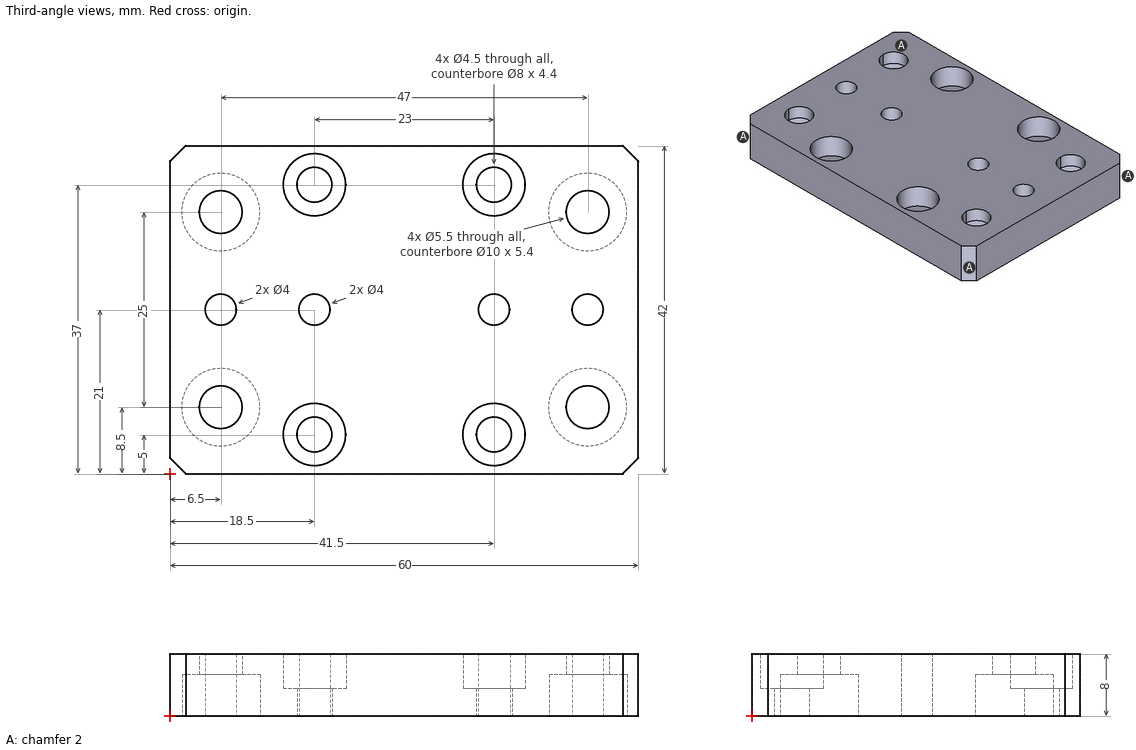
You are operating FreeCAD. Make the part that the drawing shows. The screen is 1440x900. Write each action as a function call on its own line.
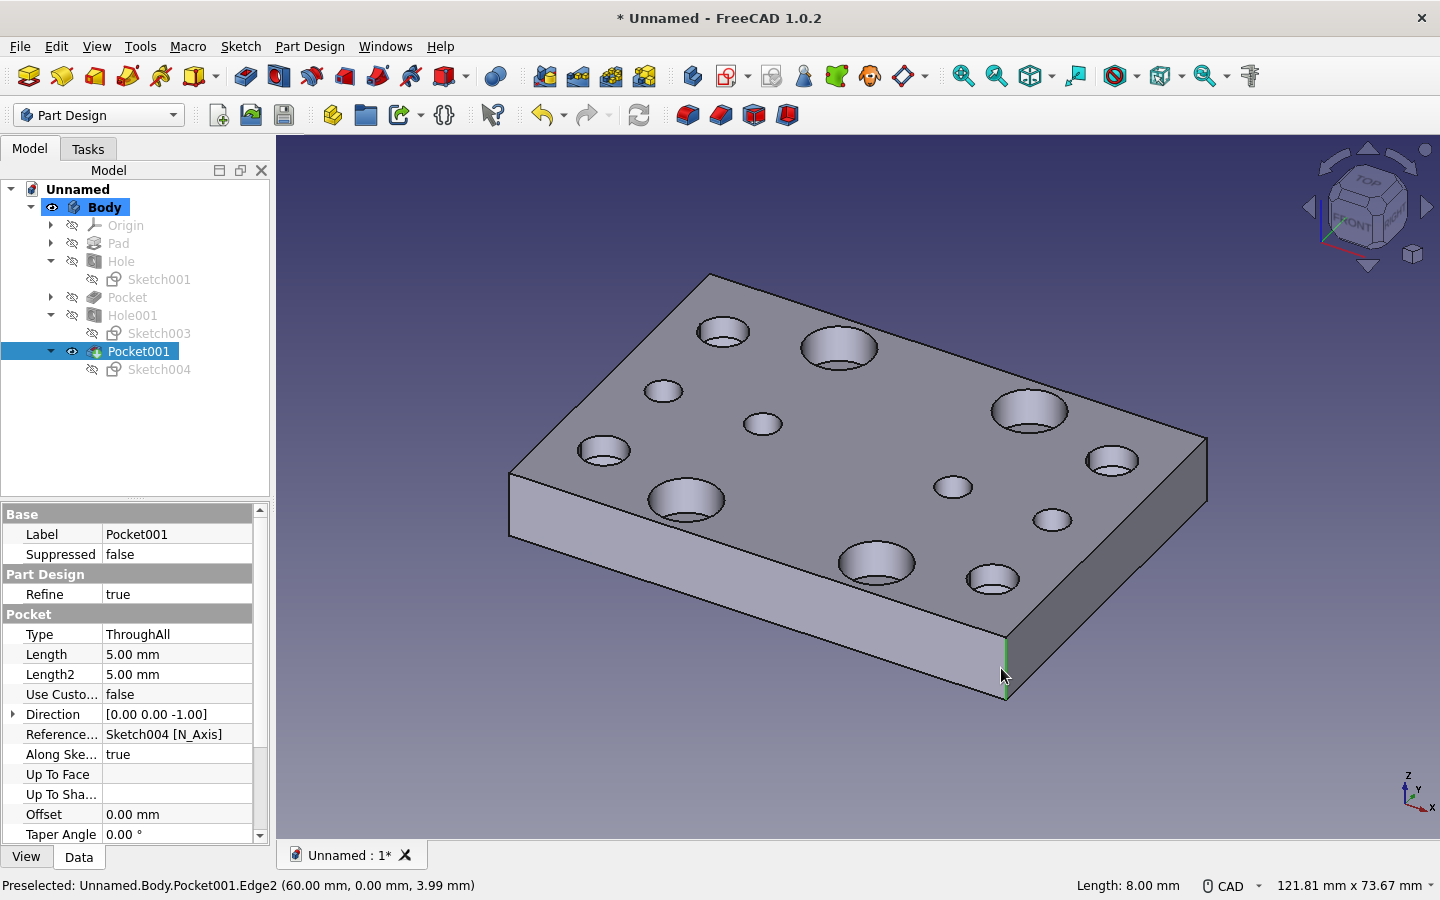
key(0)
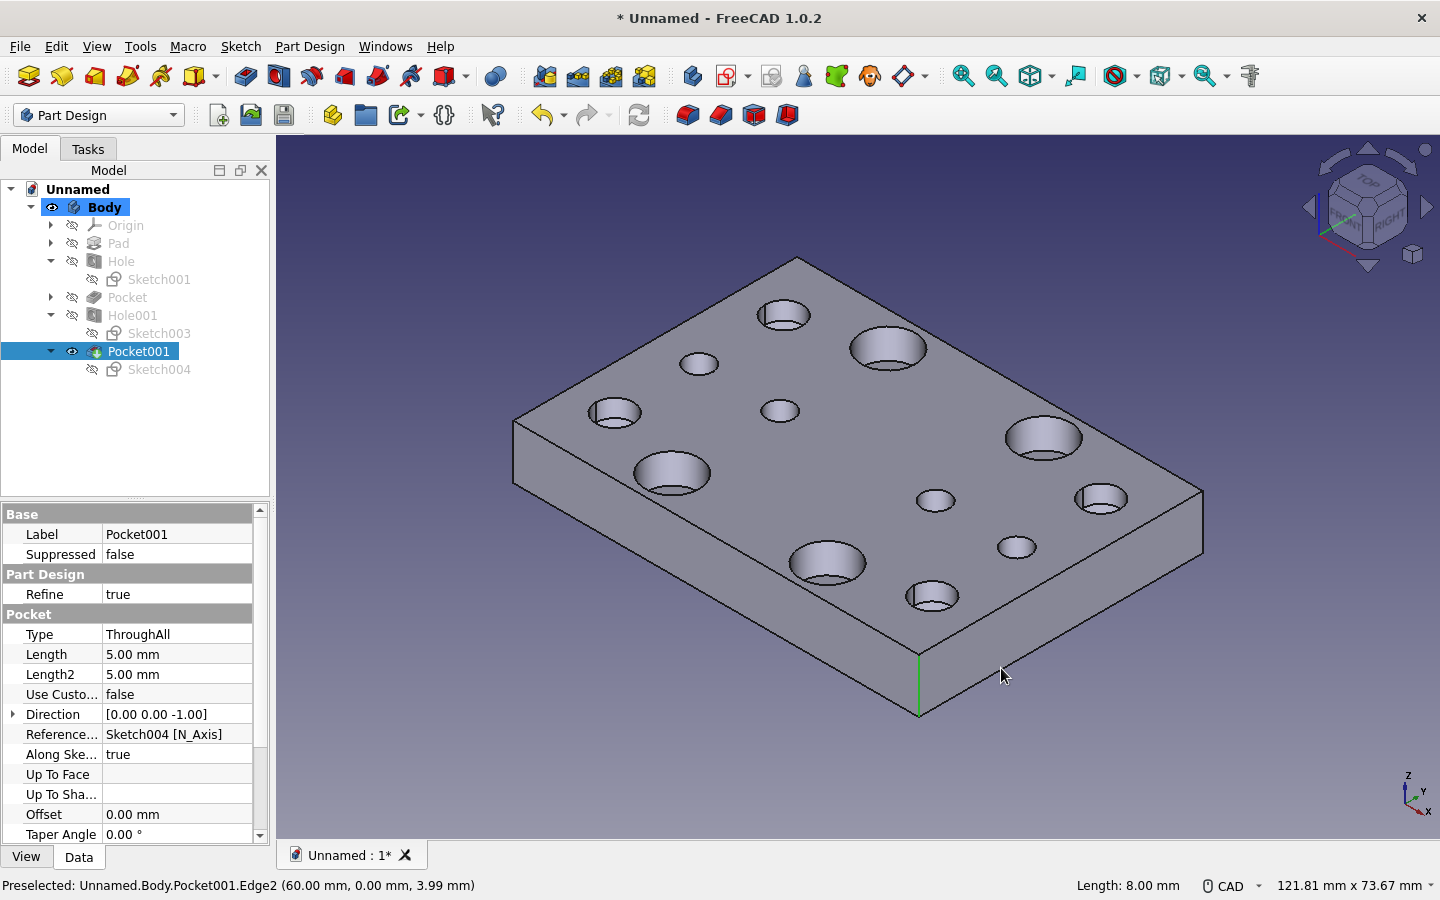
key(2)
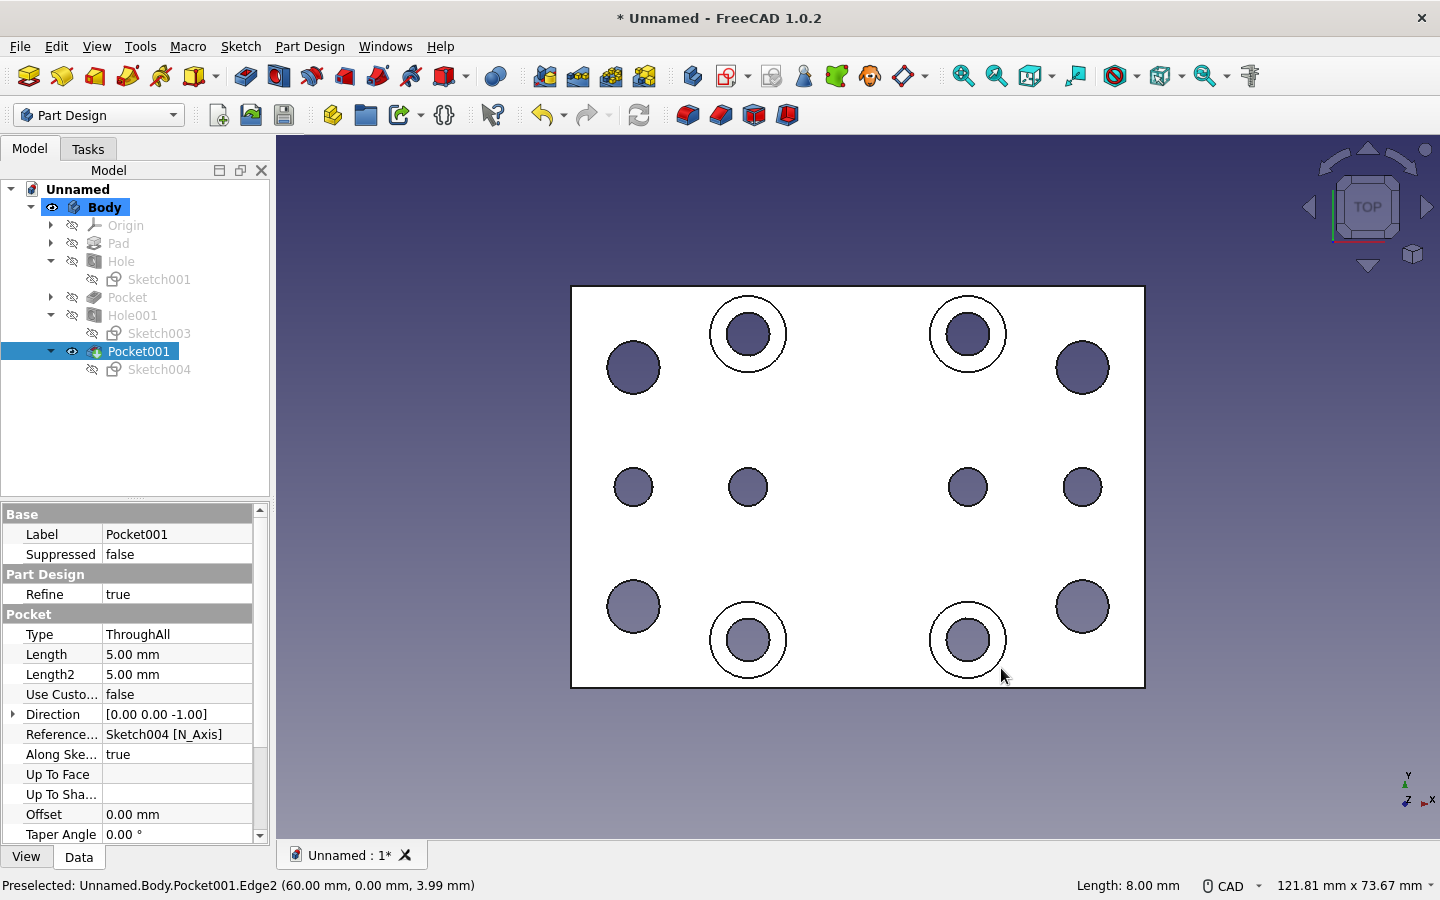
key(1)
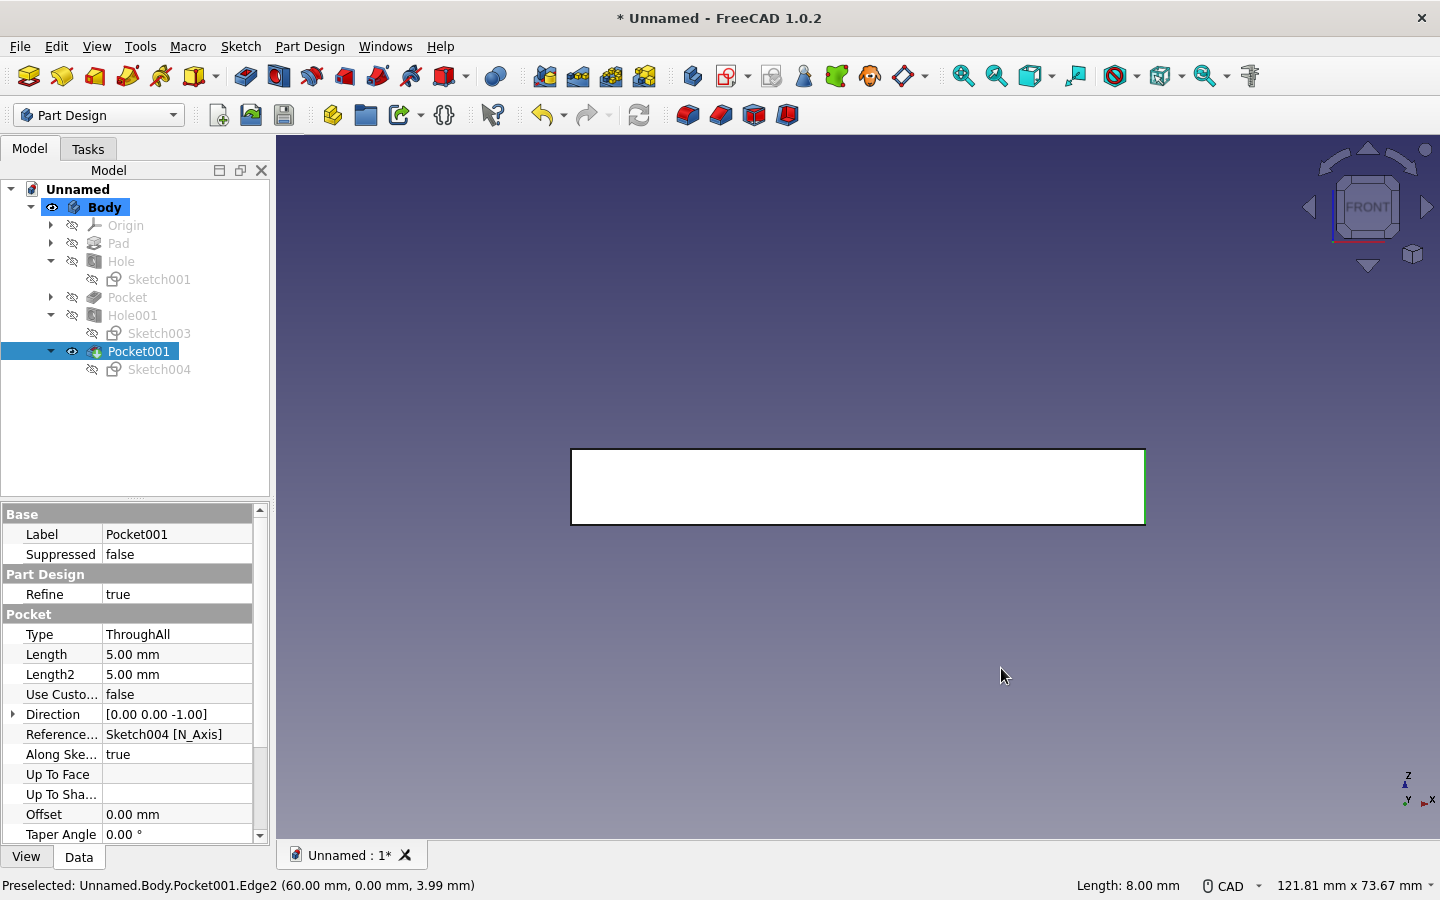
click(571, 486, ctrl)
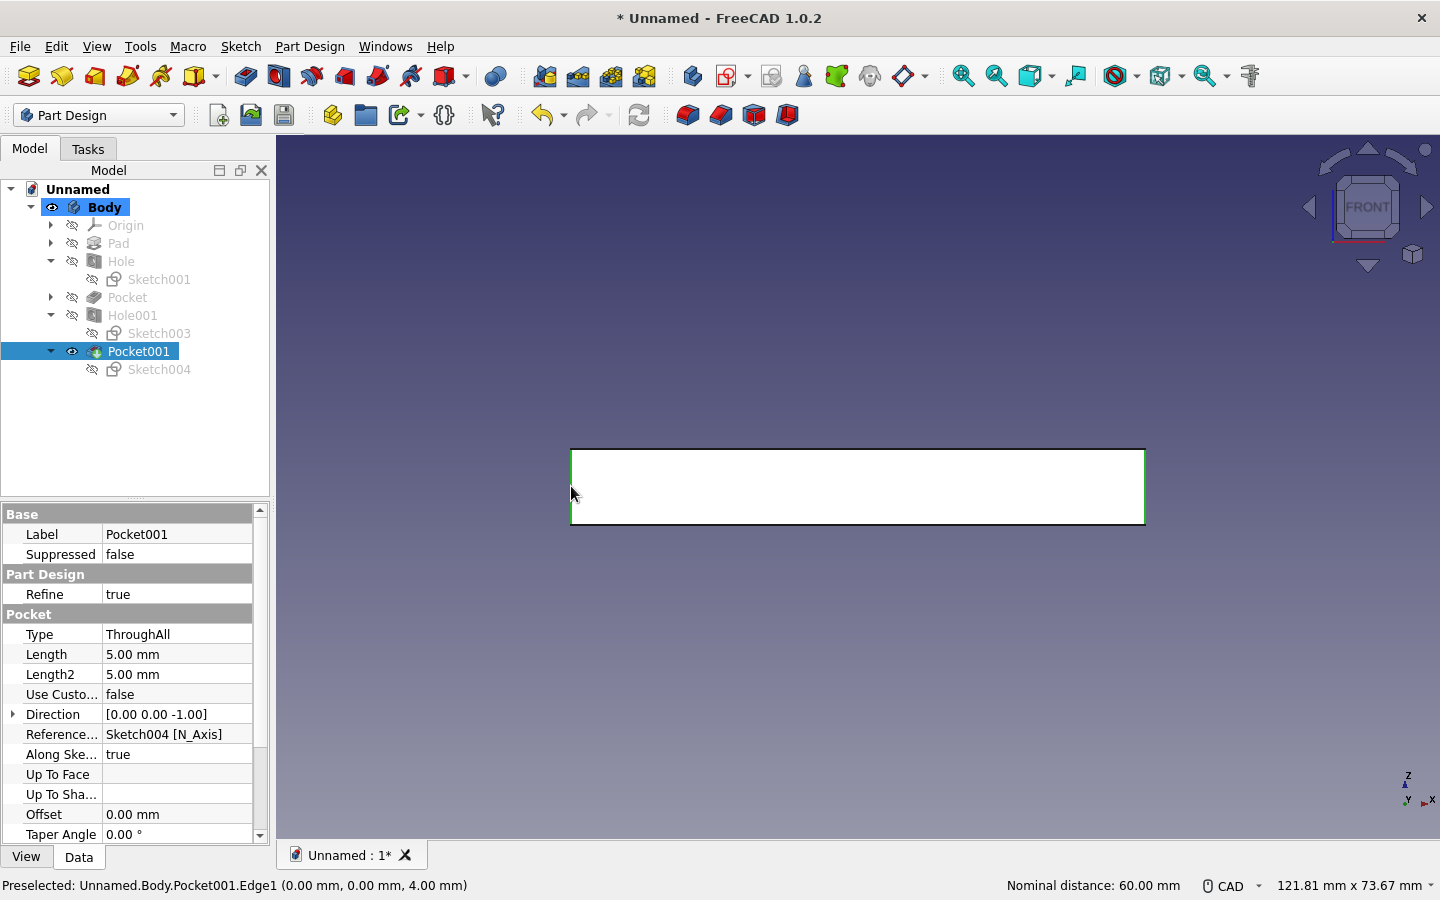
key(3)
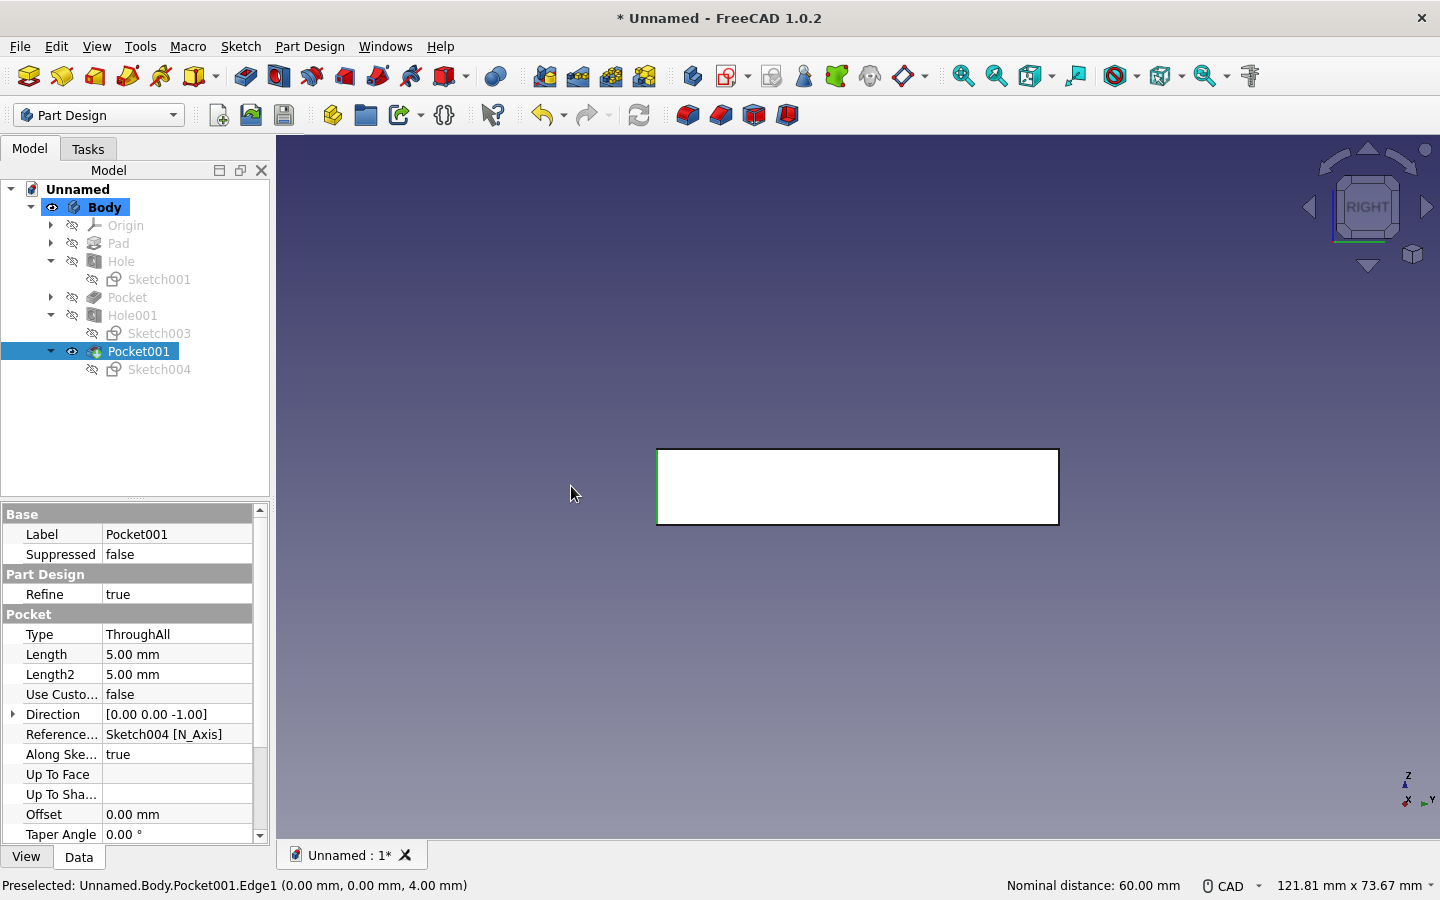
click(964, 76)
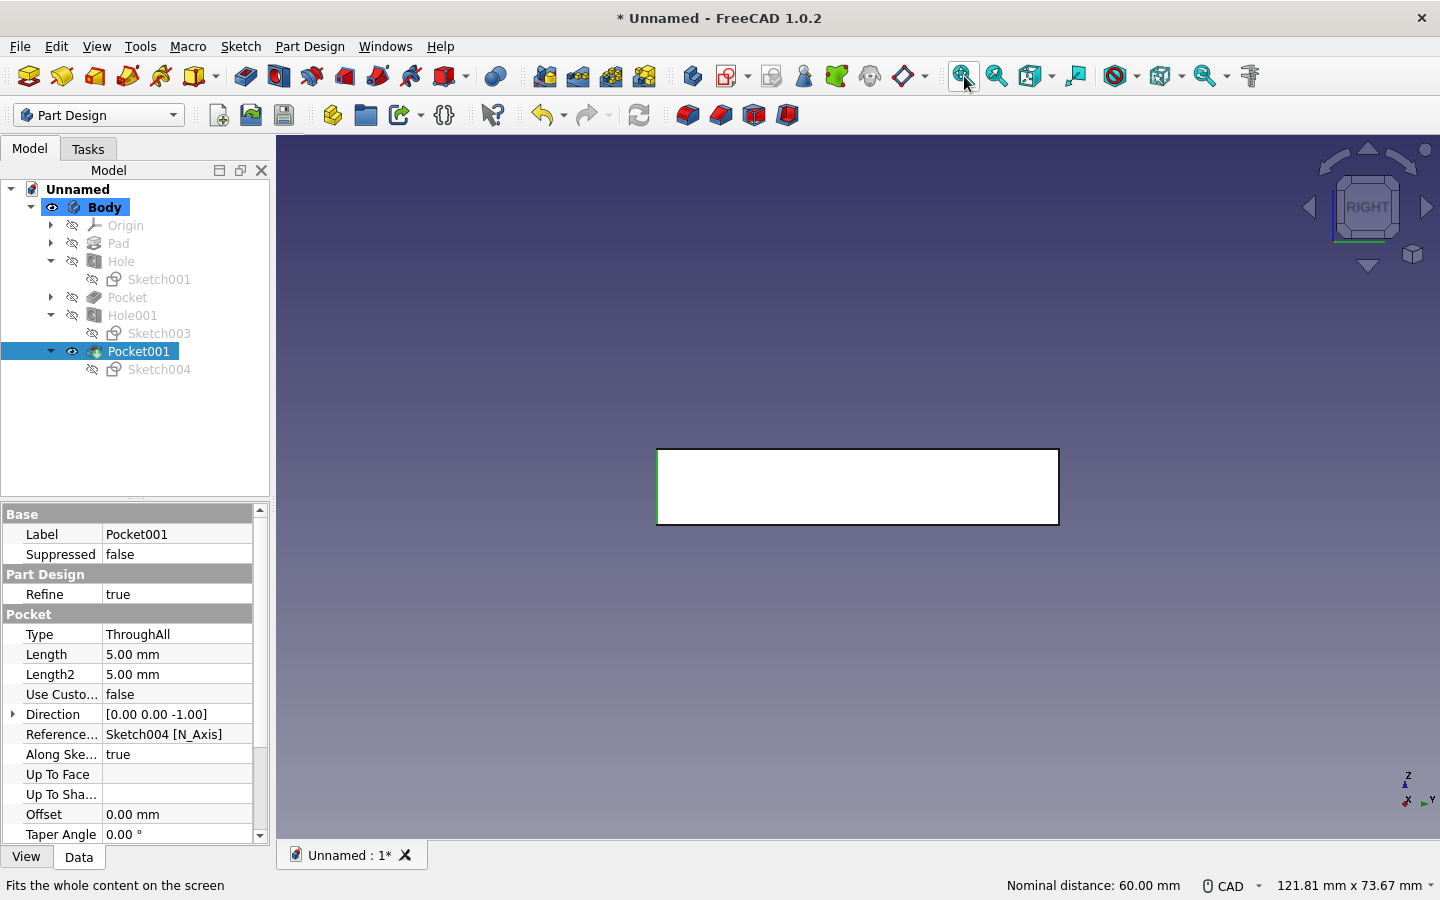
click(1059, 486, ctrl)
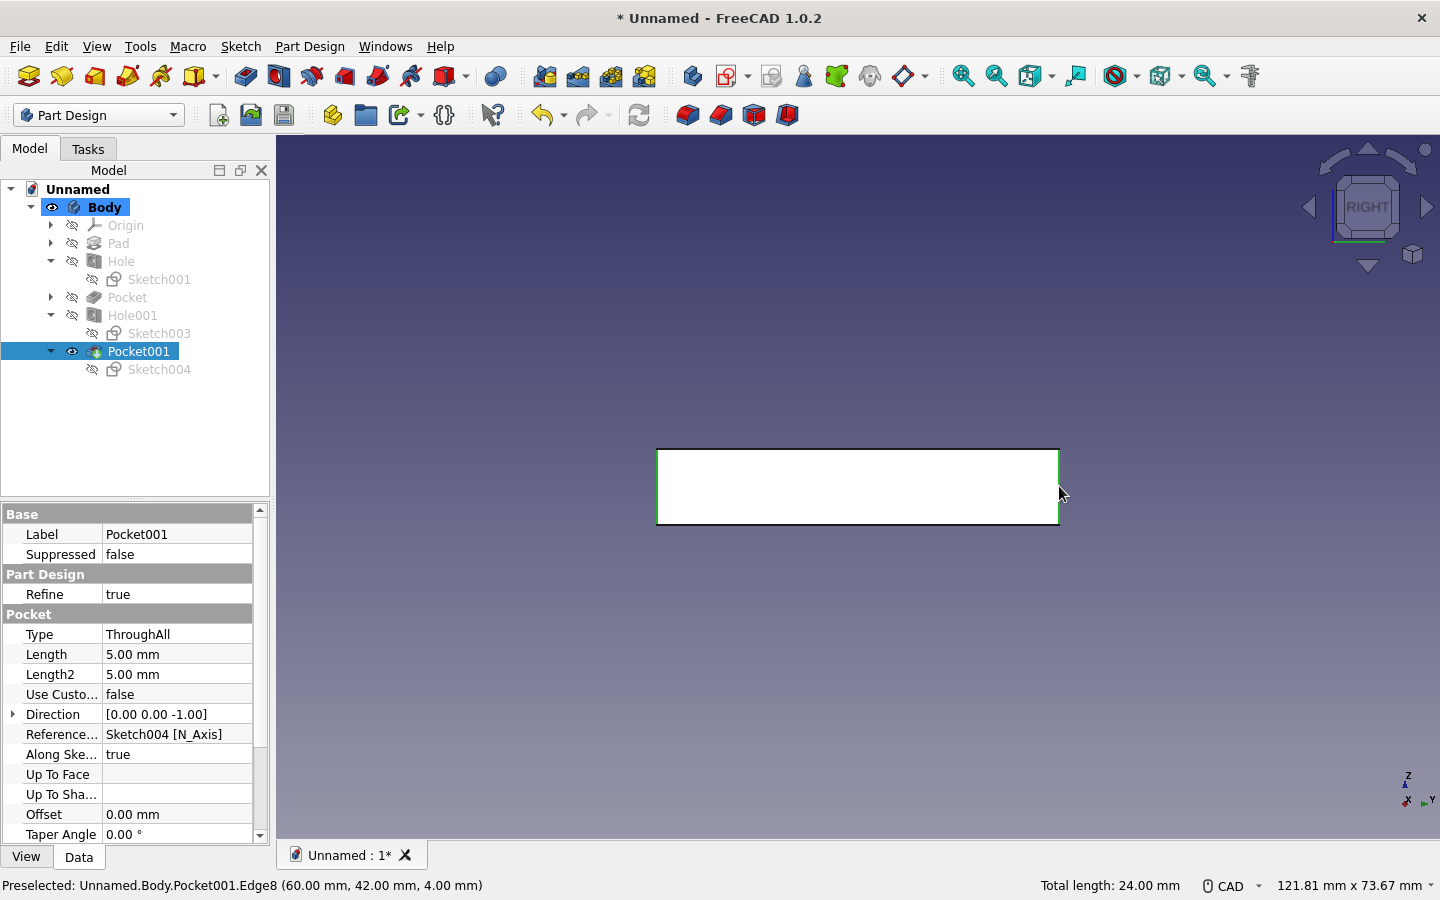
key(5)